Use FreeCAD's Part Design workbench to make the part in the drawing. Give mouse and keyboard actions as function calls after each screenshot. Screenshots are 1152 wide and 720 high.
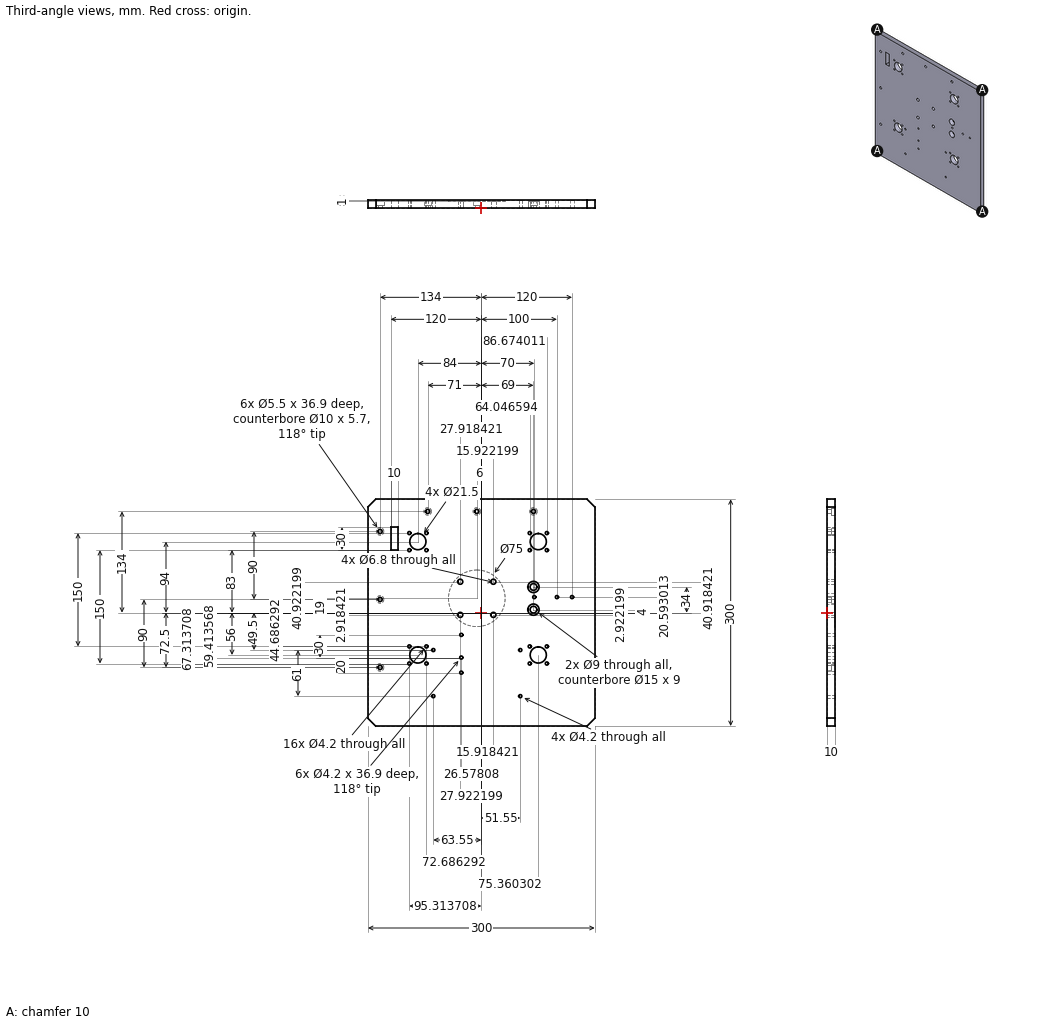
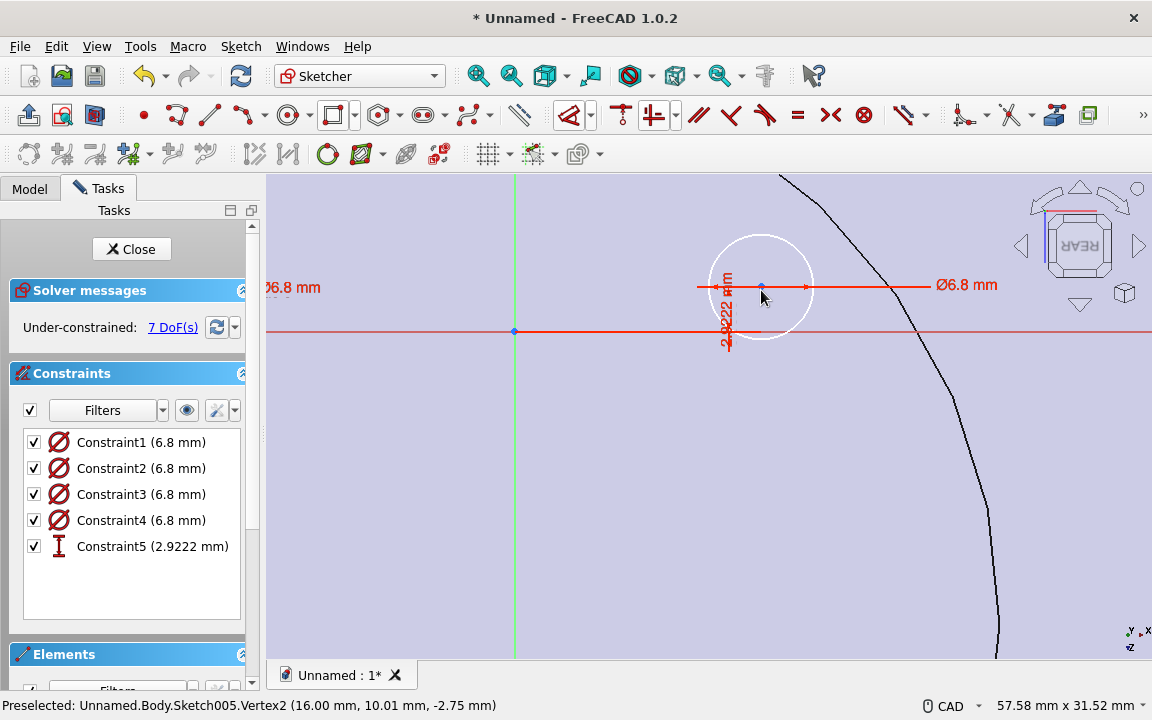
scroll(767, 296, down, 5)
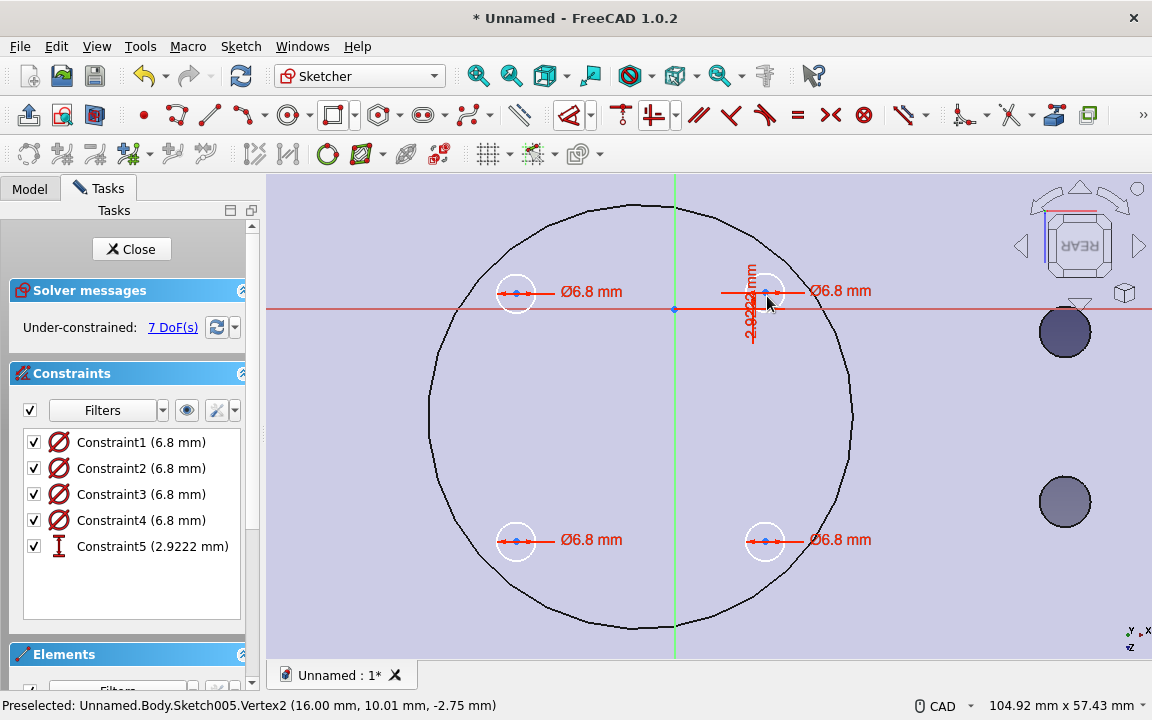
scroll(516, 294, up, 5)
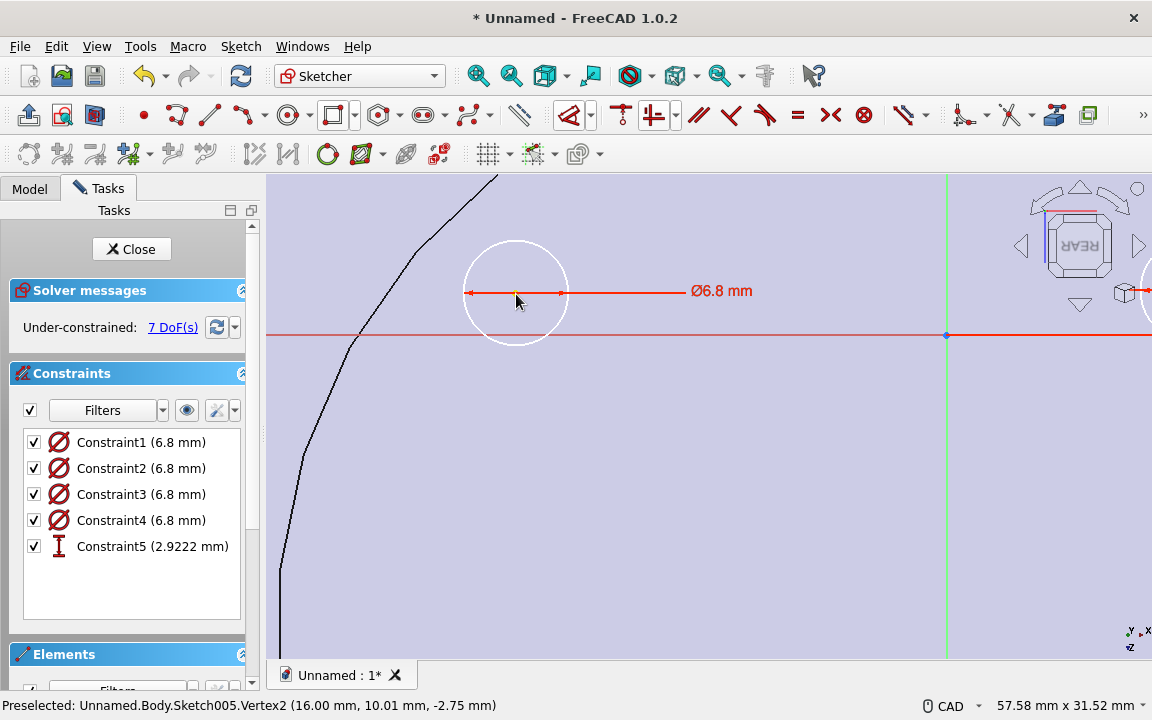
click(516, 293)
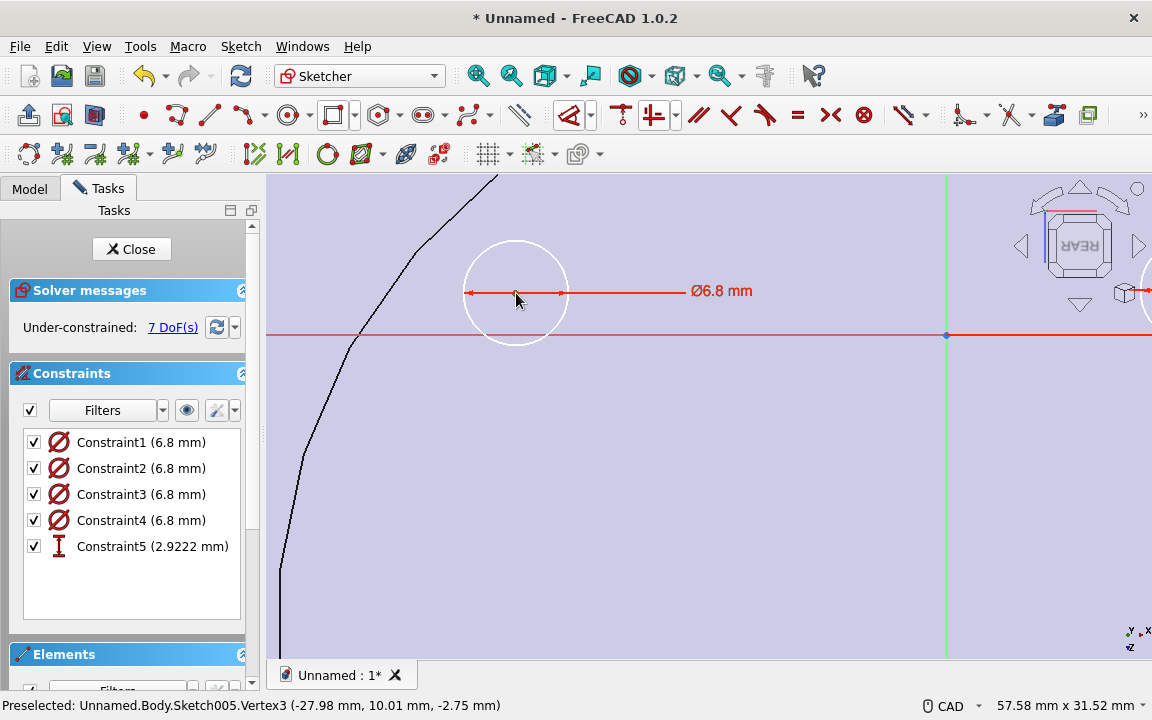
key(i)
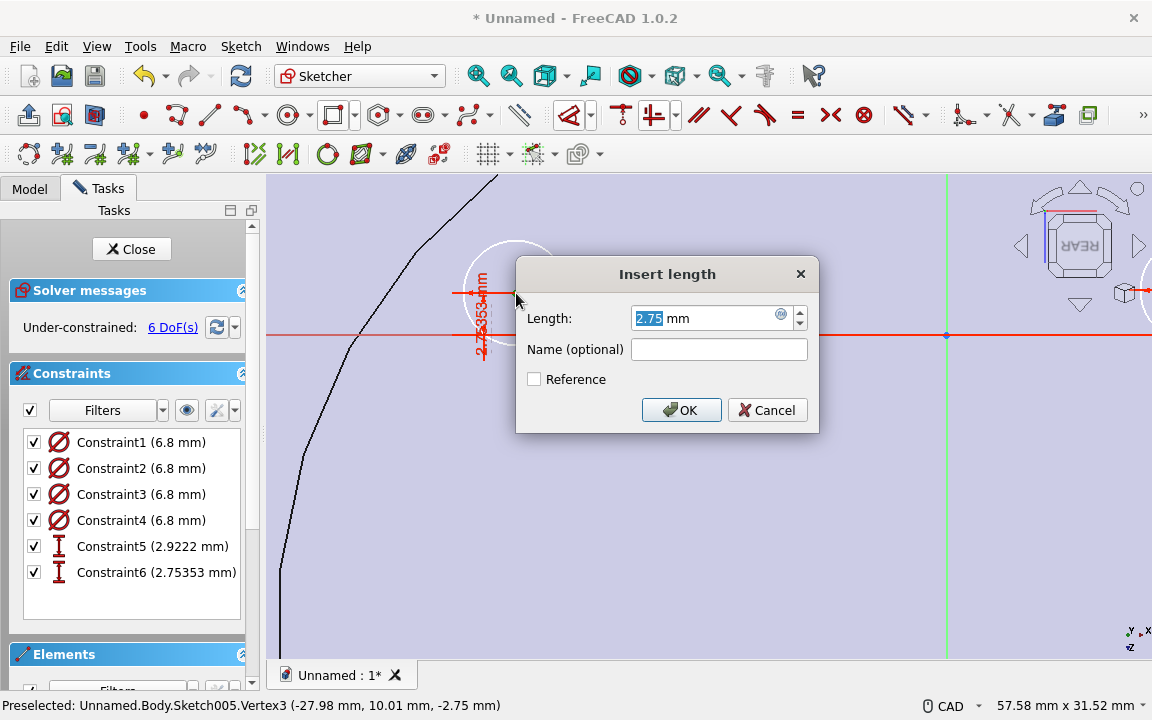
text(2.918421)
key(Return)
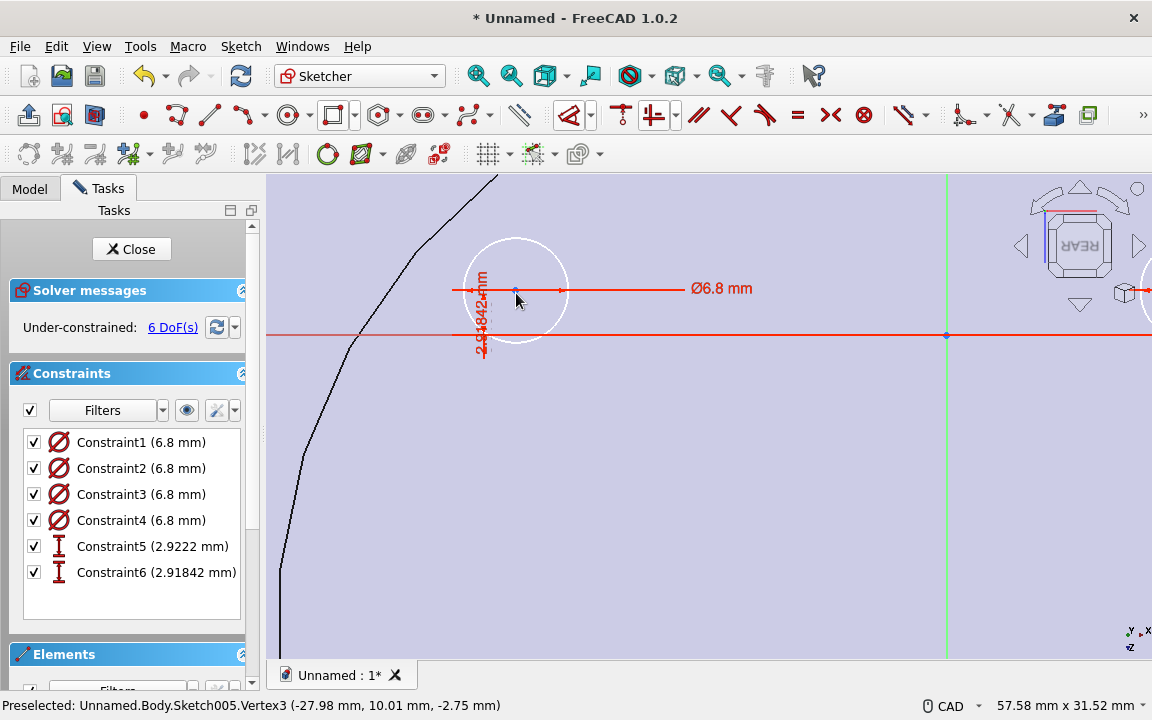
scroll(516, 294, down, 5)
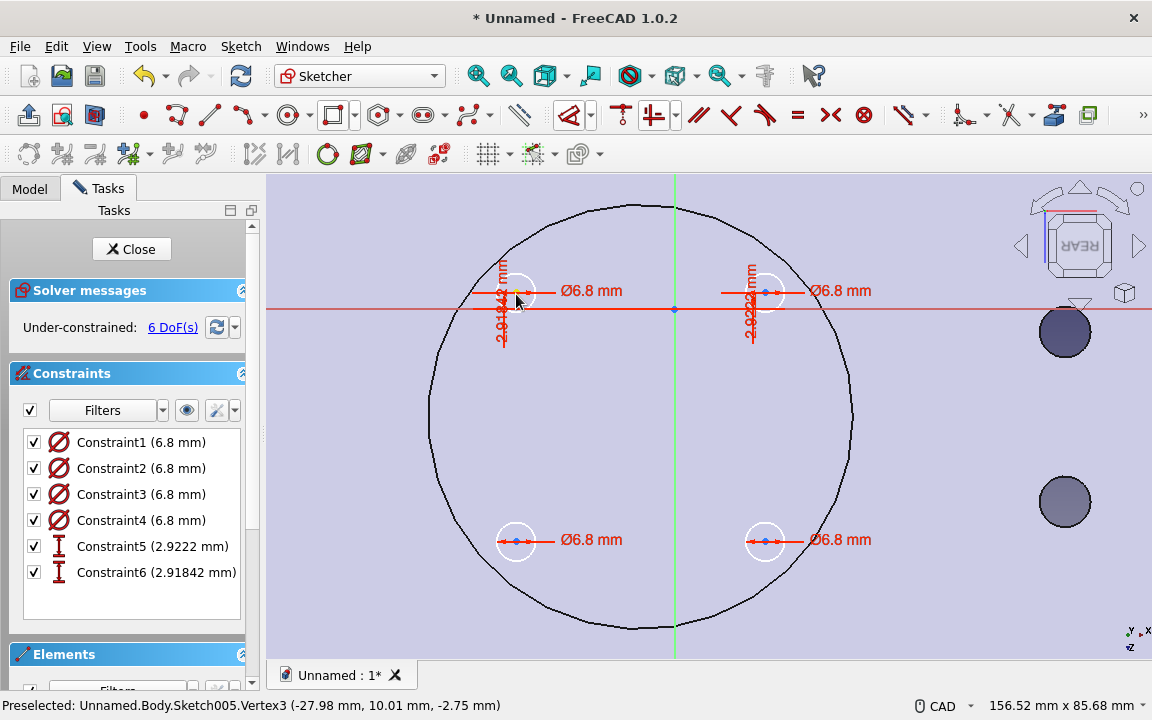
click(765, 542)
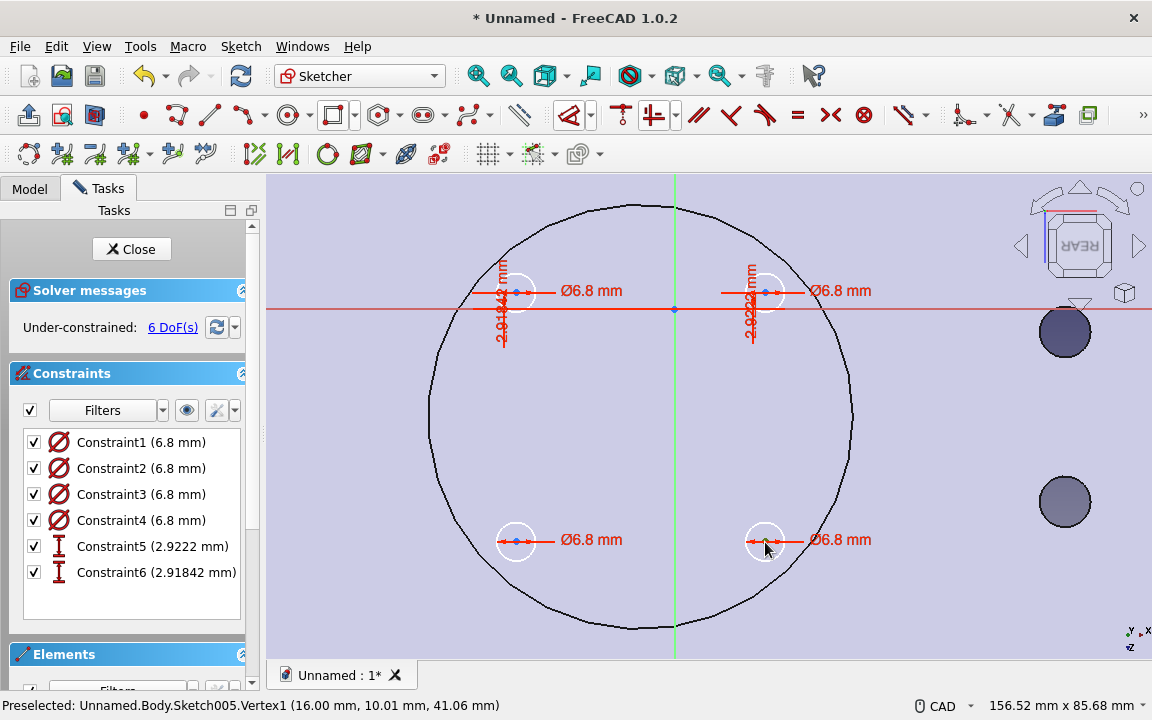
click(590, 116)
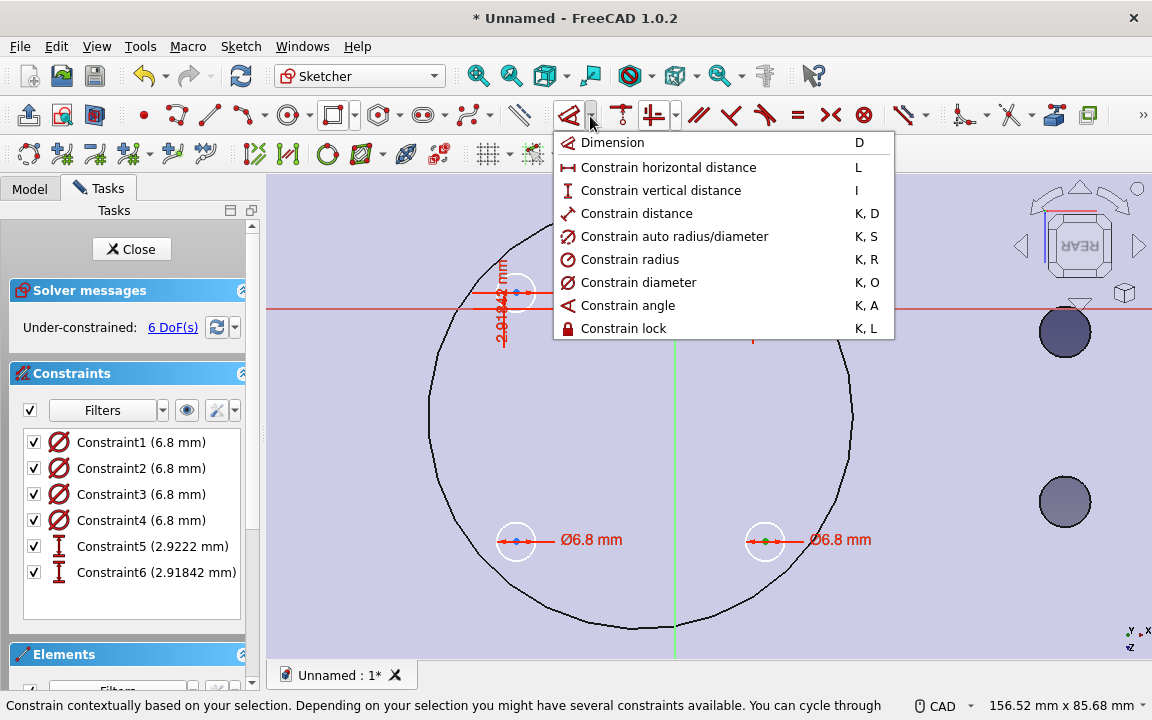
click(724, 168)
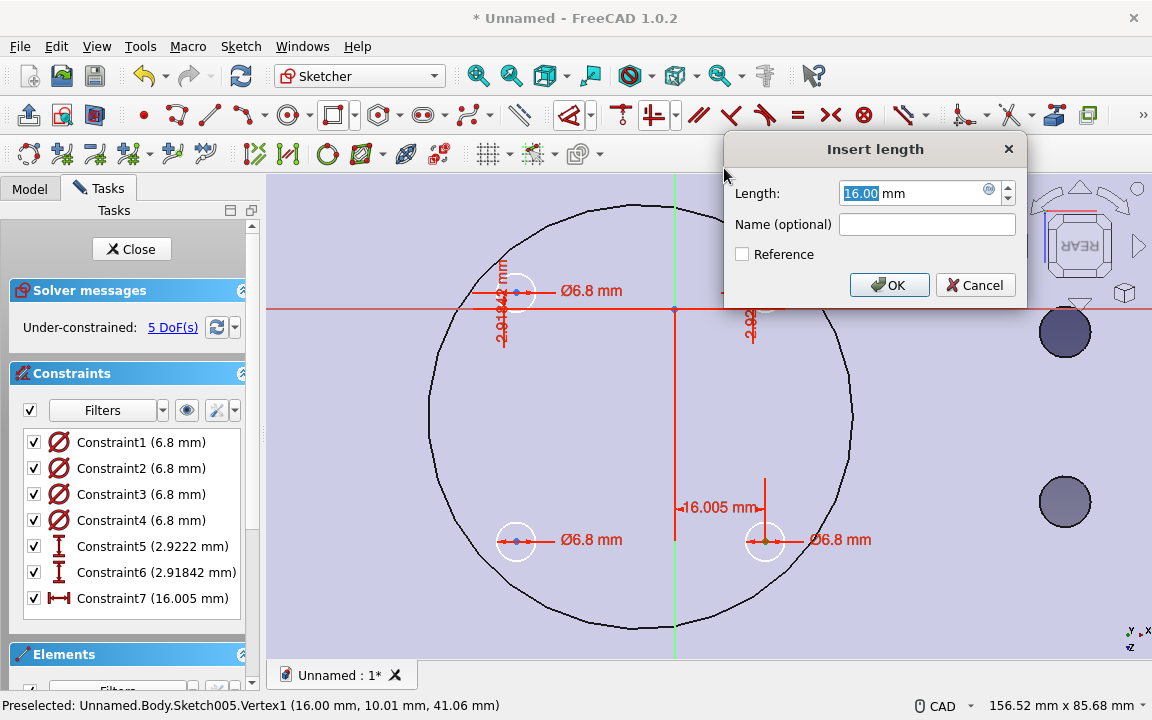
text(15.922199)
key(Return)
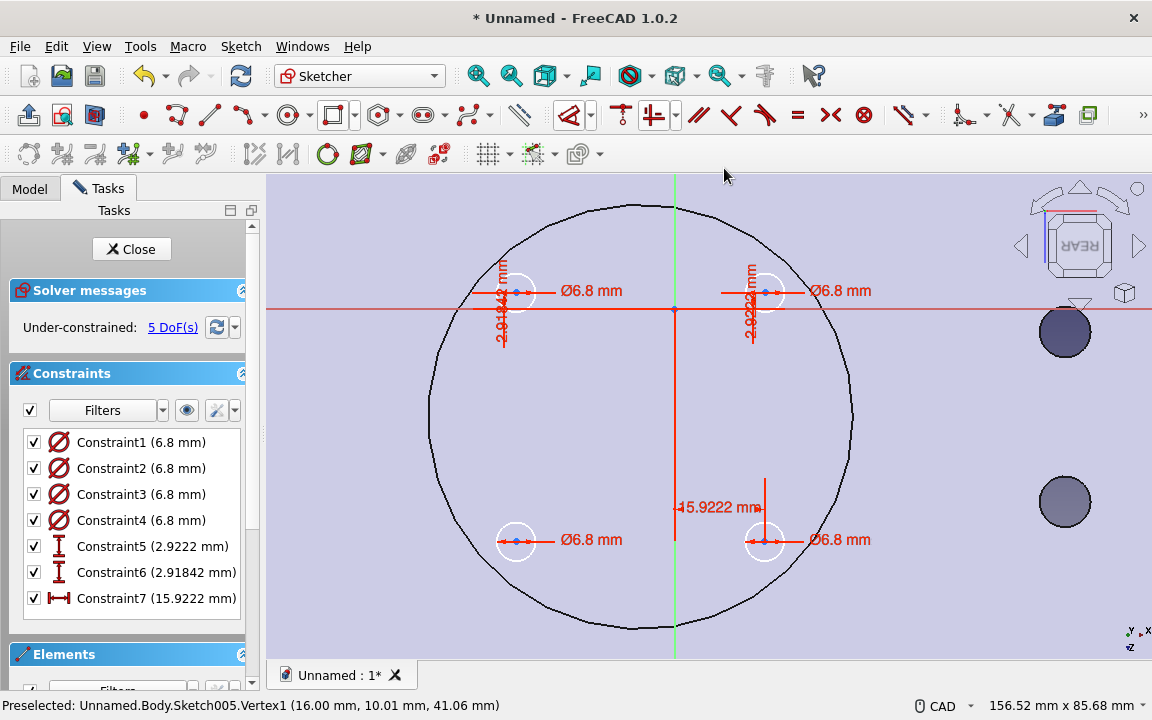
click(765, 542)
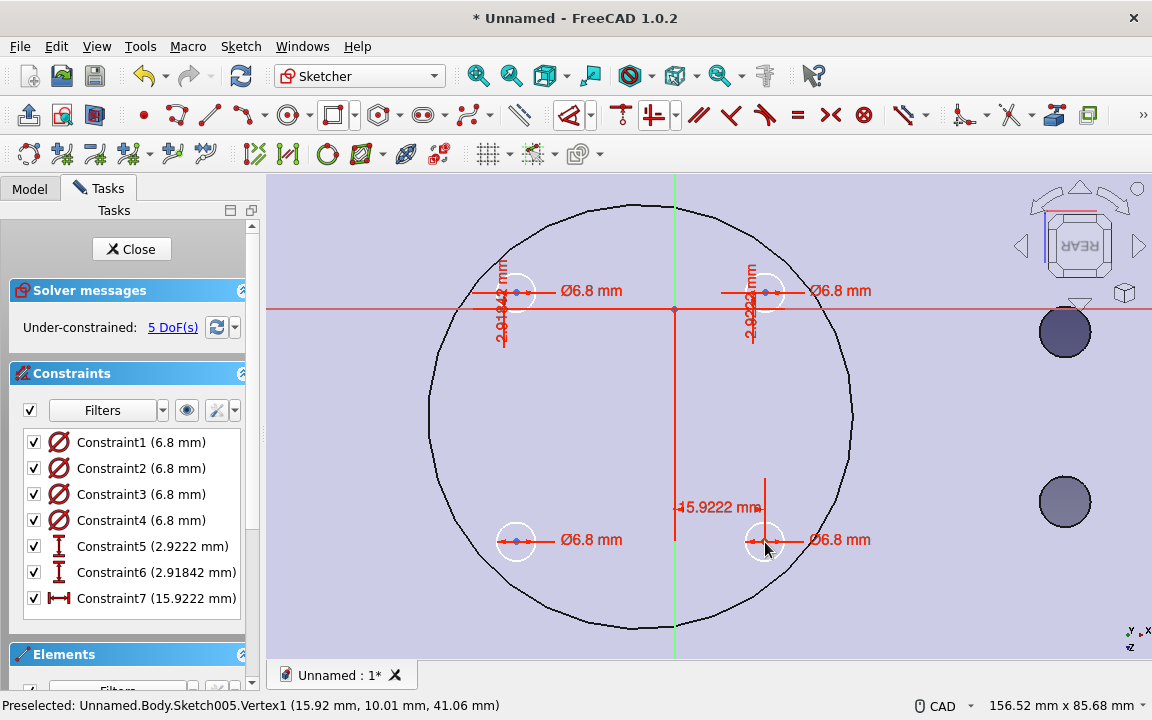
key(i)